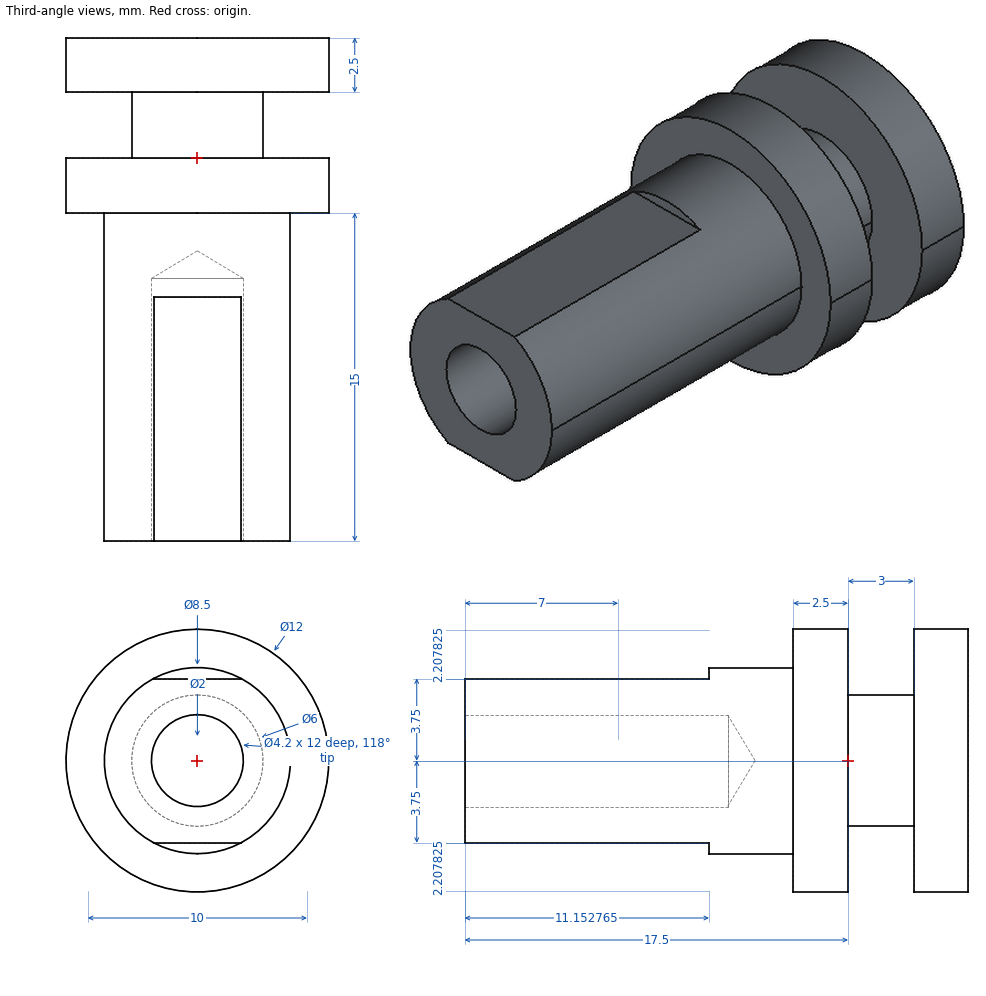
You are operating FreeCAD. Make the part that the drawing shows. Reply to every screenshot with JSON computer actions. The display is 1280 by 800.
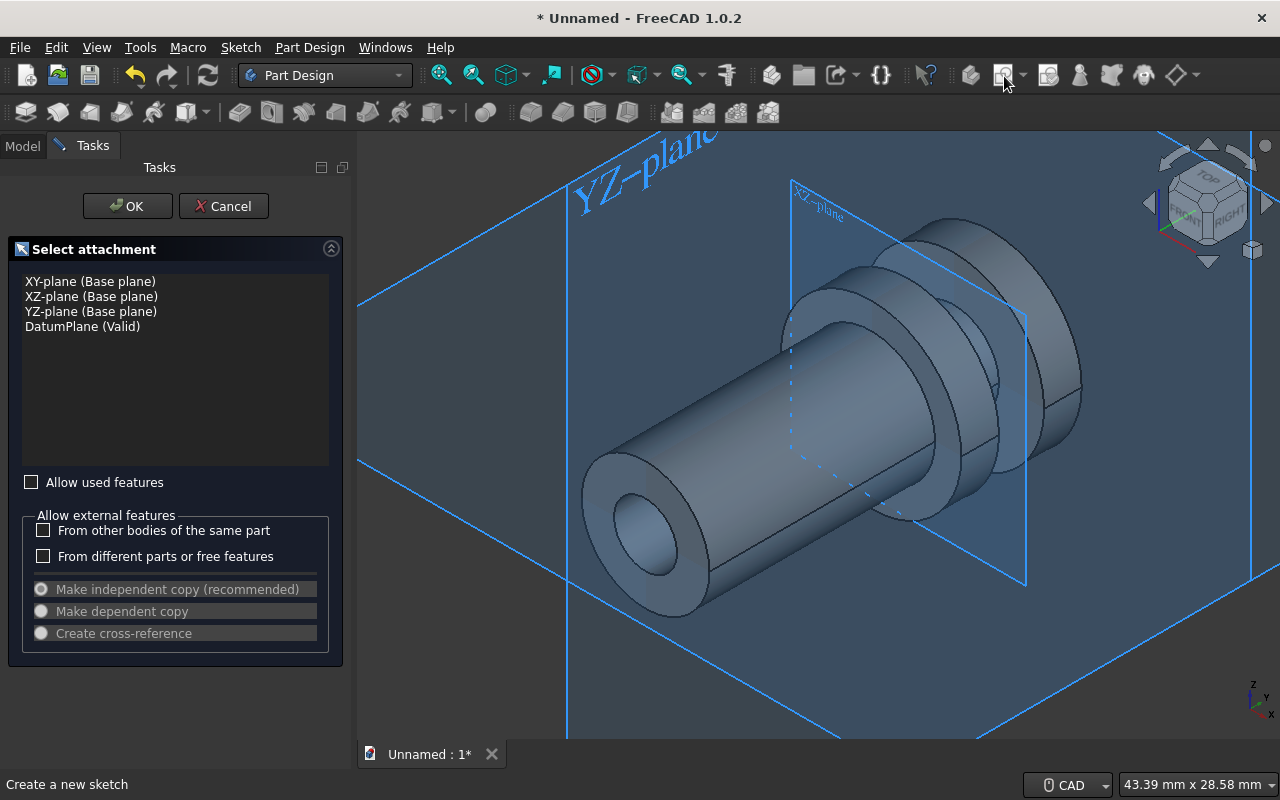
{"action": "left_click", "coordinate": [82, 312]}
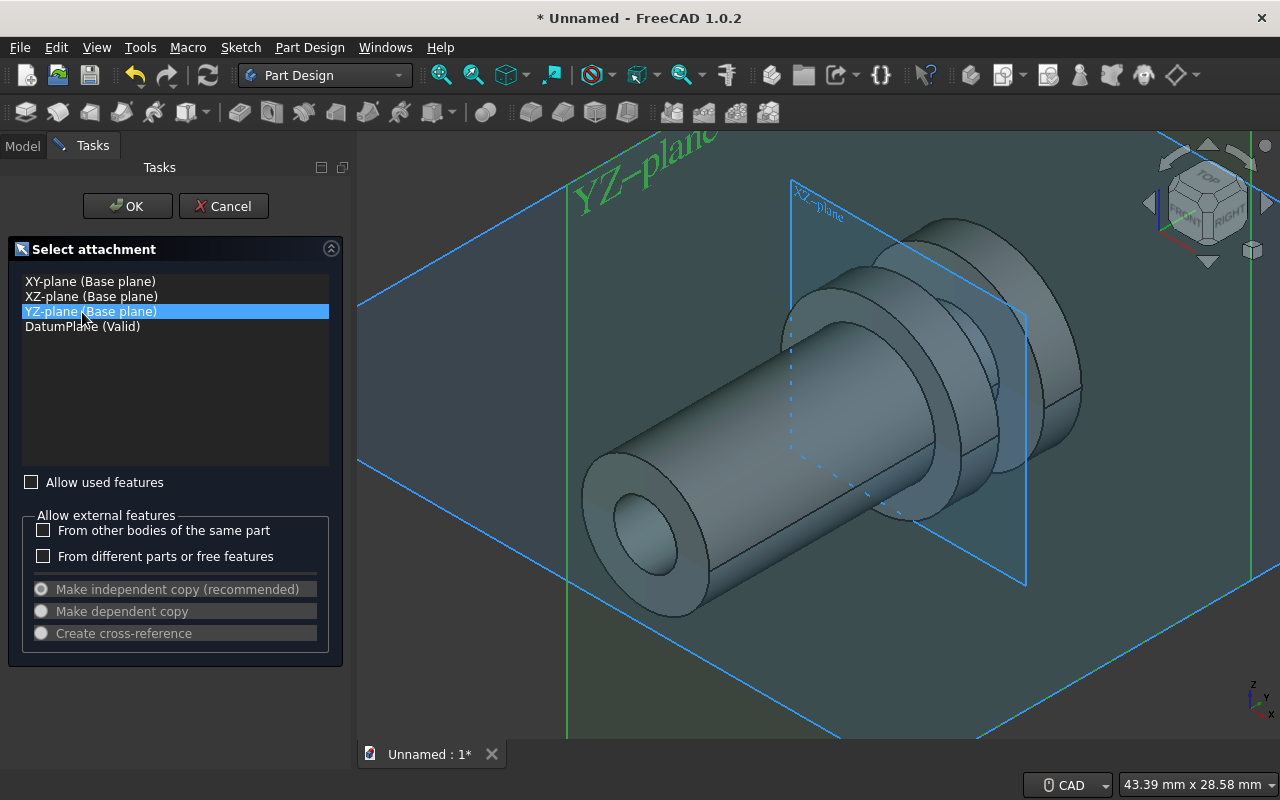
{"action": "left_click", "coordinate": [128, 206]}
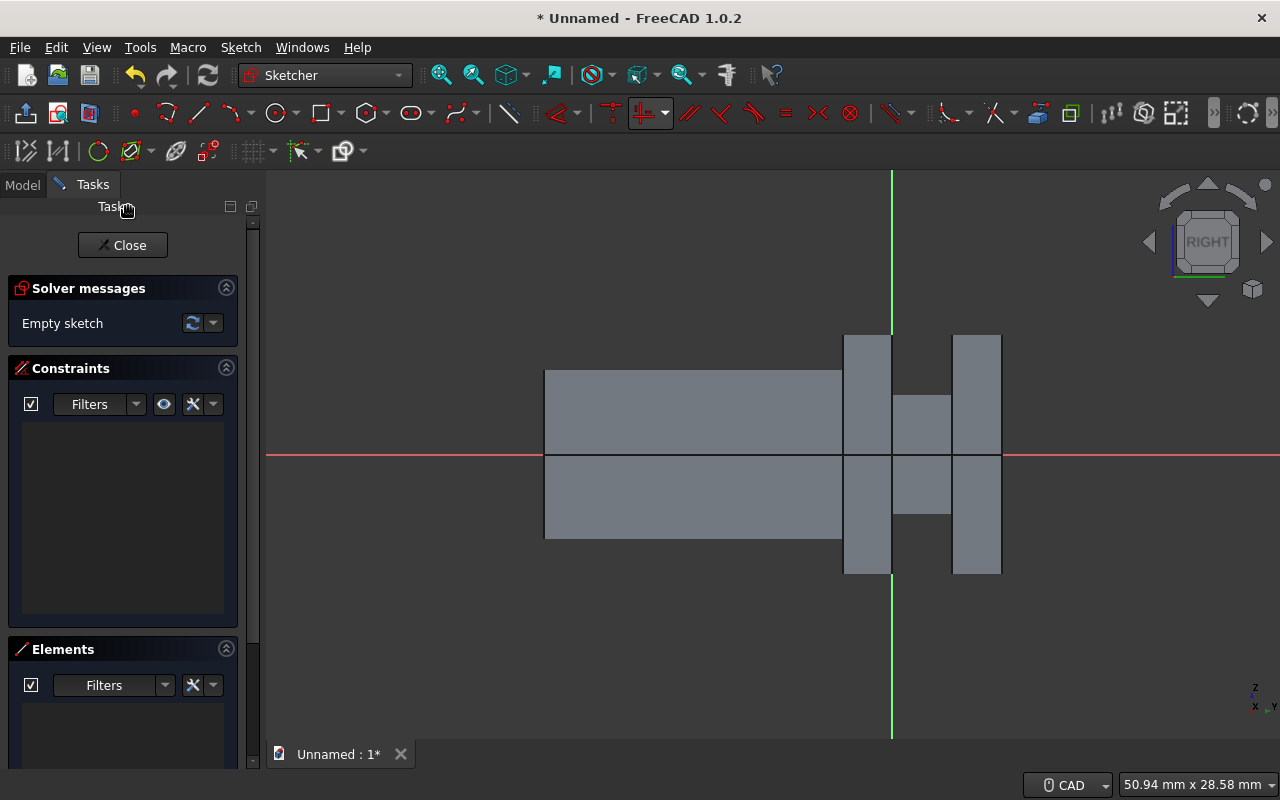
{"action": "key", "text": "q s"}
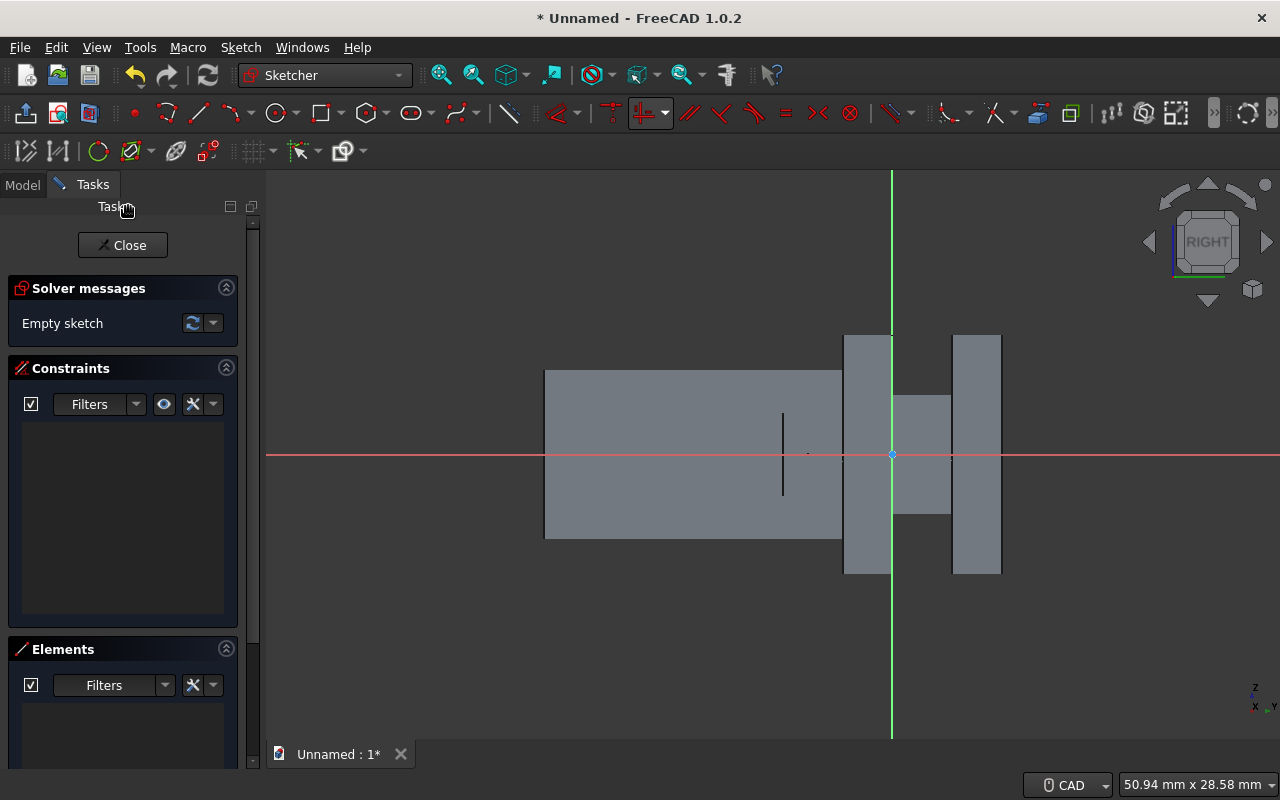
{"action": "scroll", "coordinate": [746, 454], "scroll_direction": "up", "scroll_amount": 2}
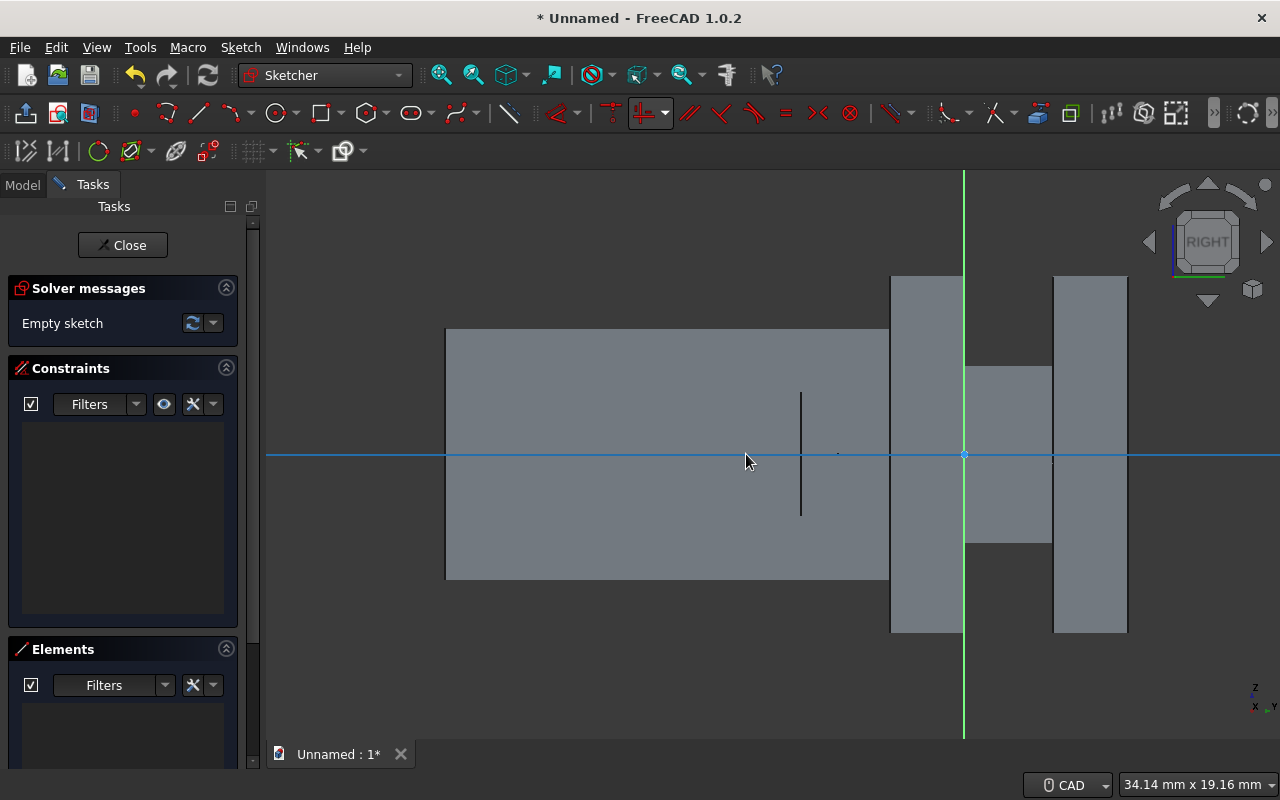
{"action": "key", "text": "g r"}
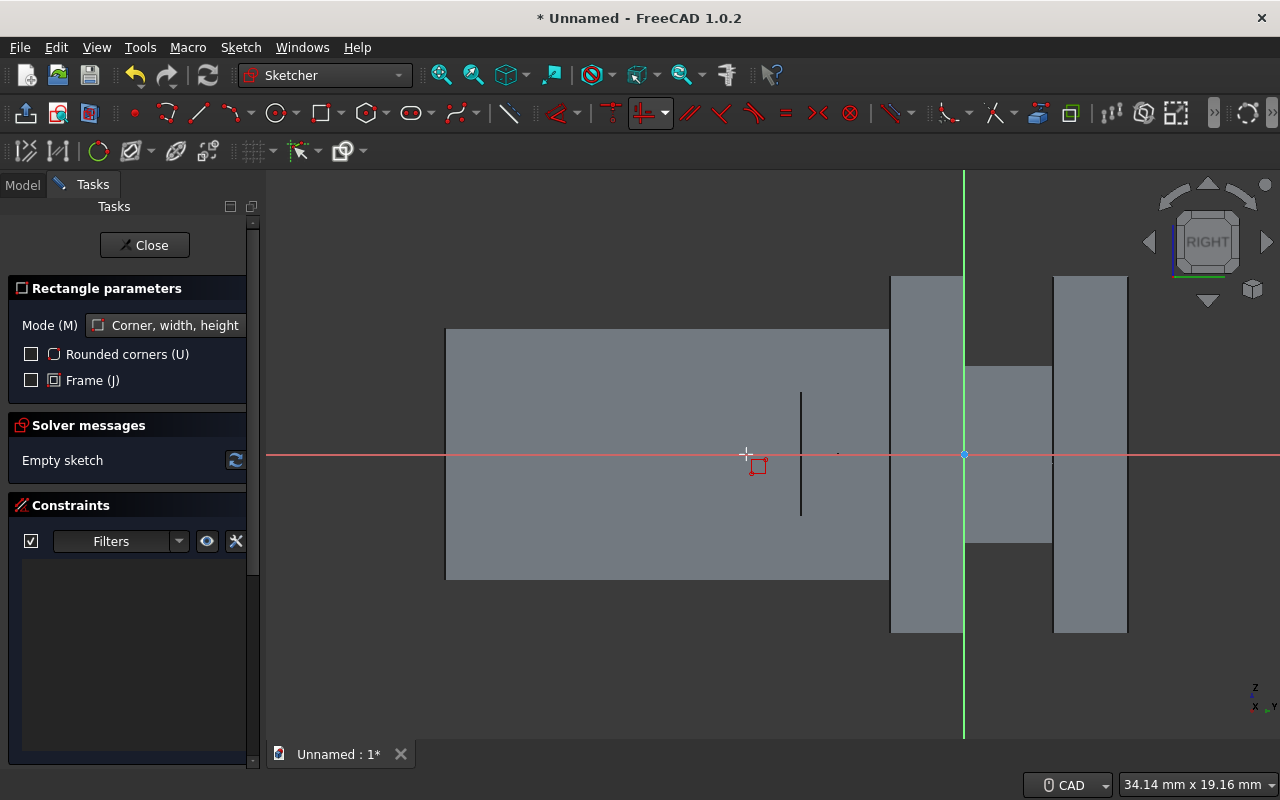
{"action": "left_click", "coordinate": [445, 566]}
{"action": "mouse_move", "coordinate": [776, 631]}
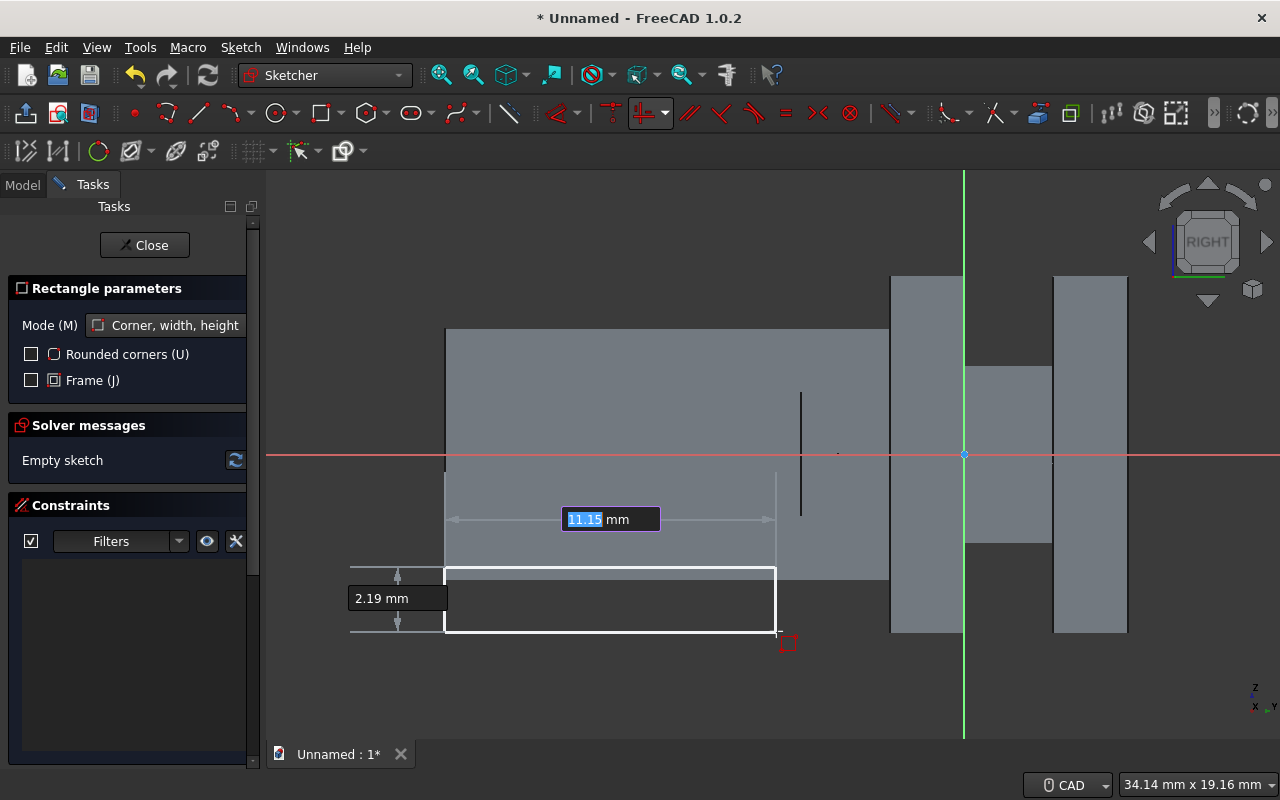
{"action": "type", "text": "11.152765"}
{"action": "key", "text": "Tab"}
{"action": "type", "text": "2.207825"}
{"action": "key", "text": "Return"}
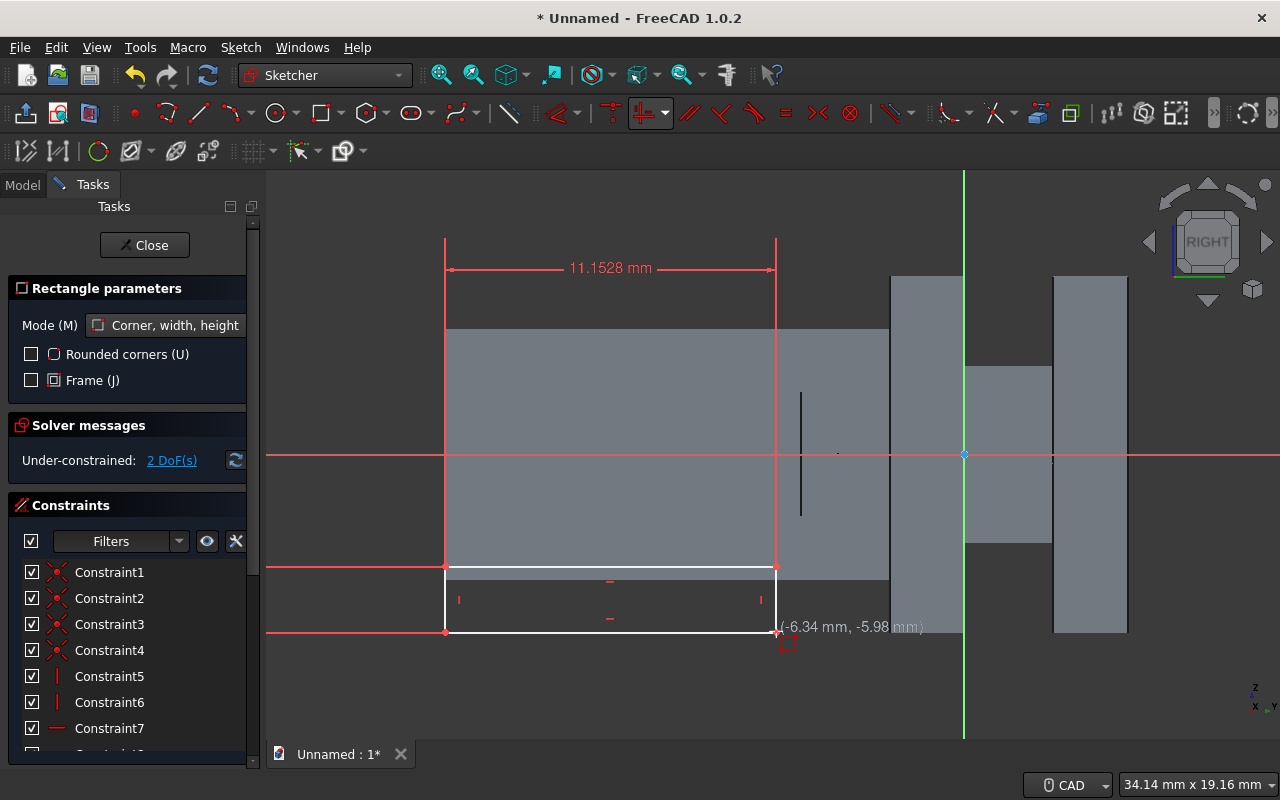
{"action": "left_click", "coordinate": [445, 278]}
{"action": "mouse_move", "coordinate": [776, 343]}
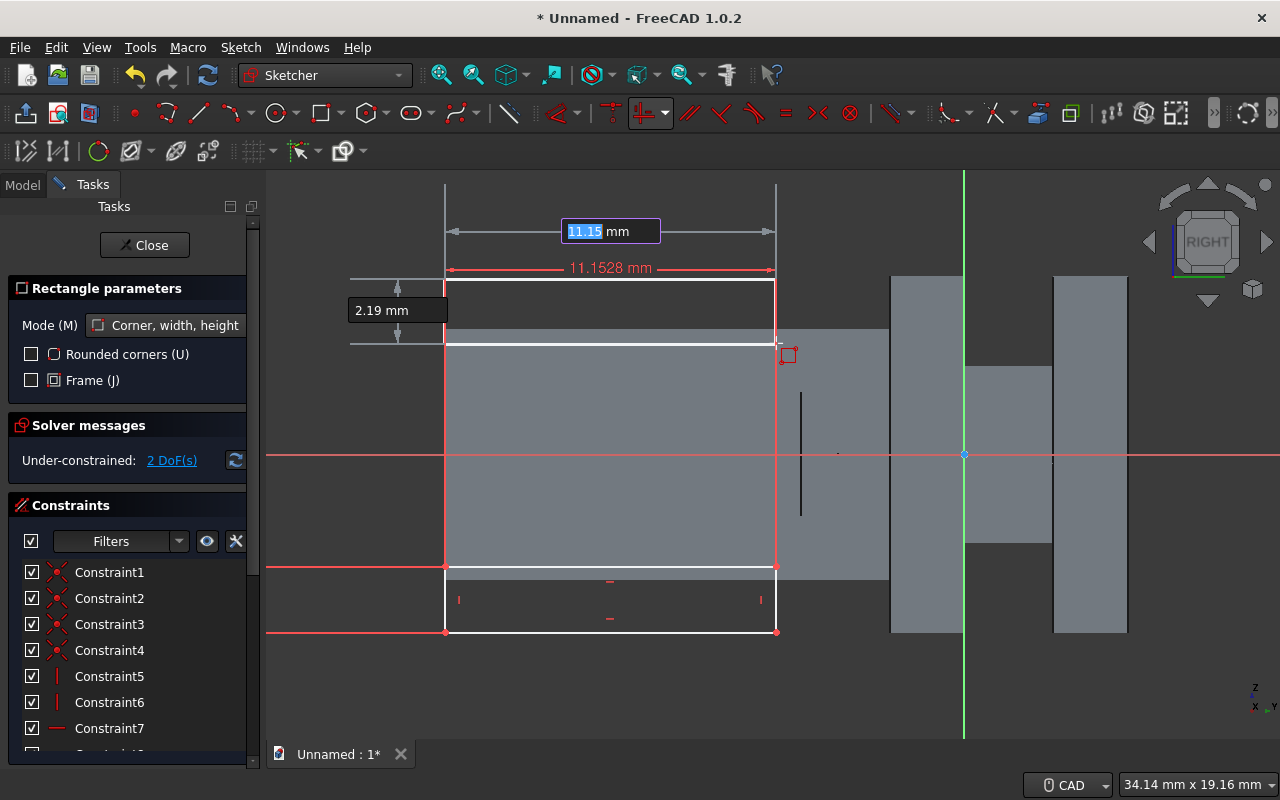
{"action": "type", "text": "11.152765"}
{"action": "key", "text": "Tab"}
{"action": "type", "text": "2.207825"}
{"action": "key", "text": "Return"}
{"action": "key", "text": "Escape"}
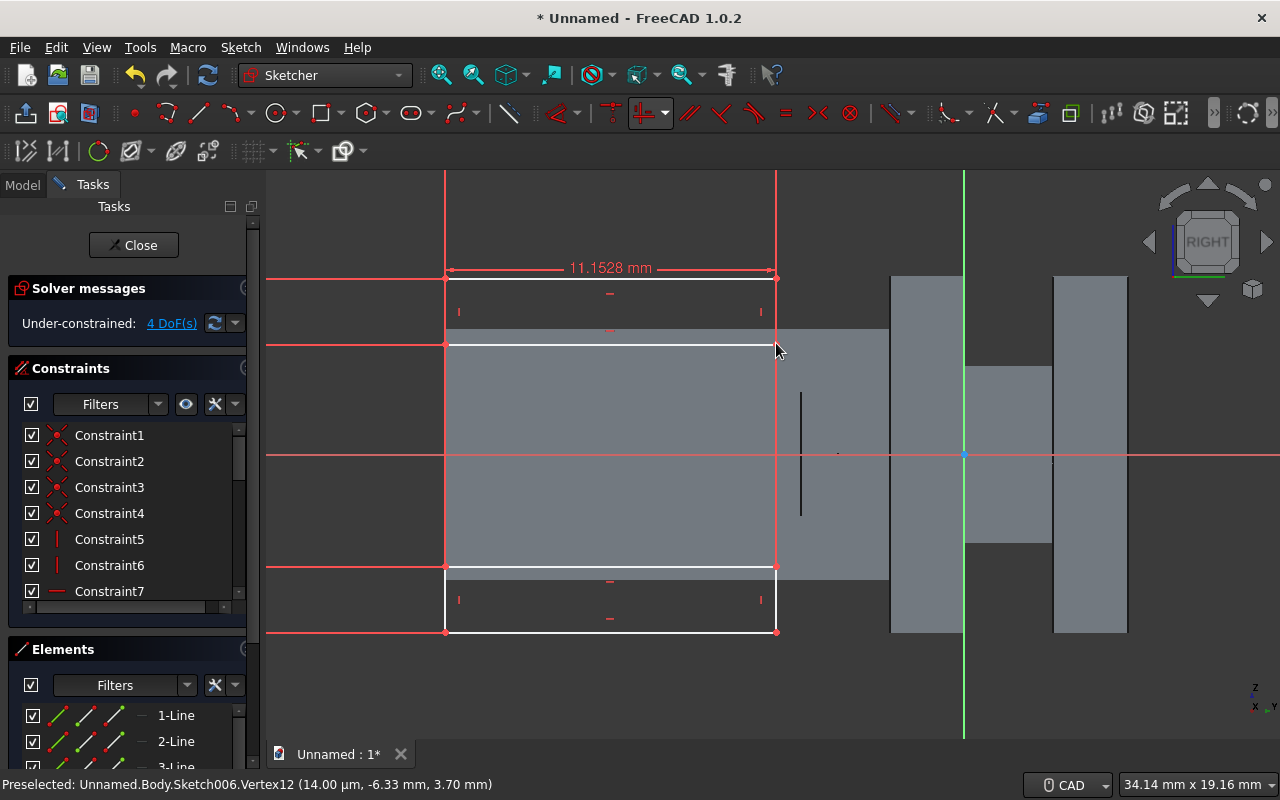
{"action": "left_click", "coordinate": [556, 114]}